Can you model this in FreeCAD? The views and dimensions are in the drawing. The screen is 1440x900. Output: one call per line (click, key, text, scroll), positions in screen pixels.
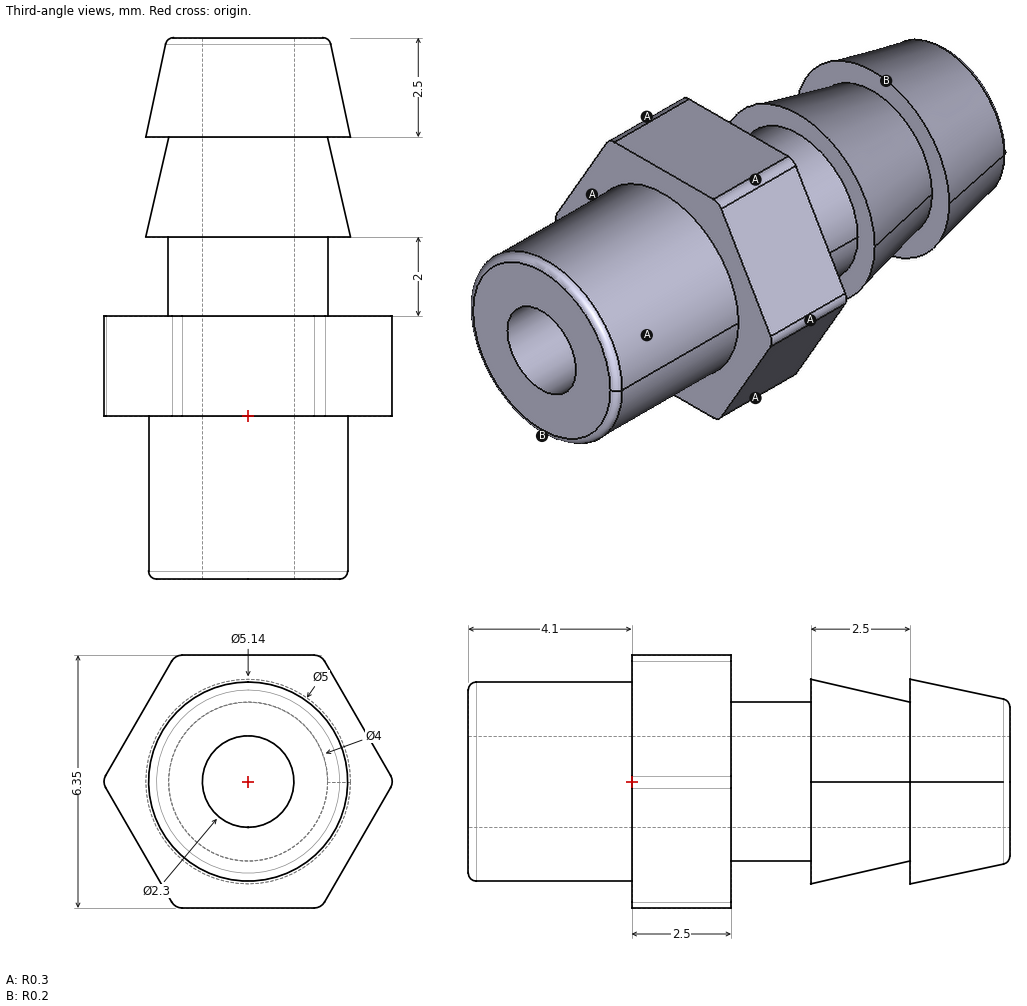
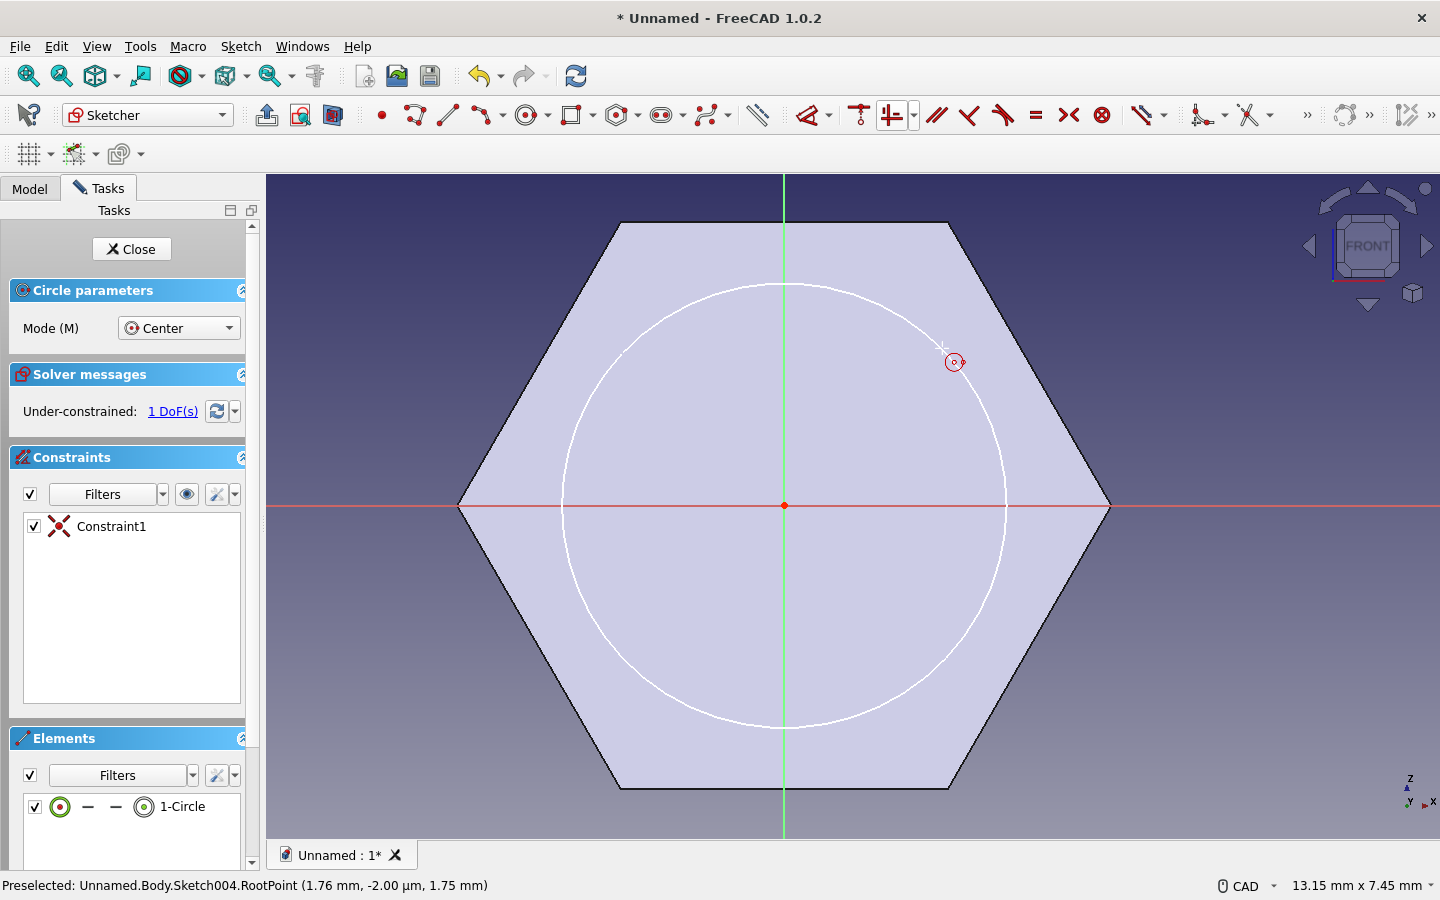
click(784, 506)
click(857, 433)
key(Escape)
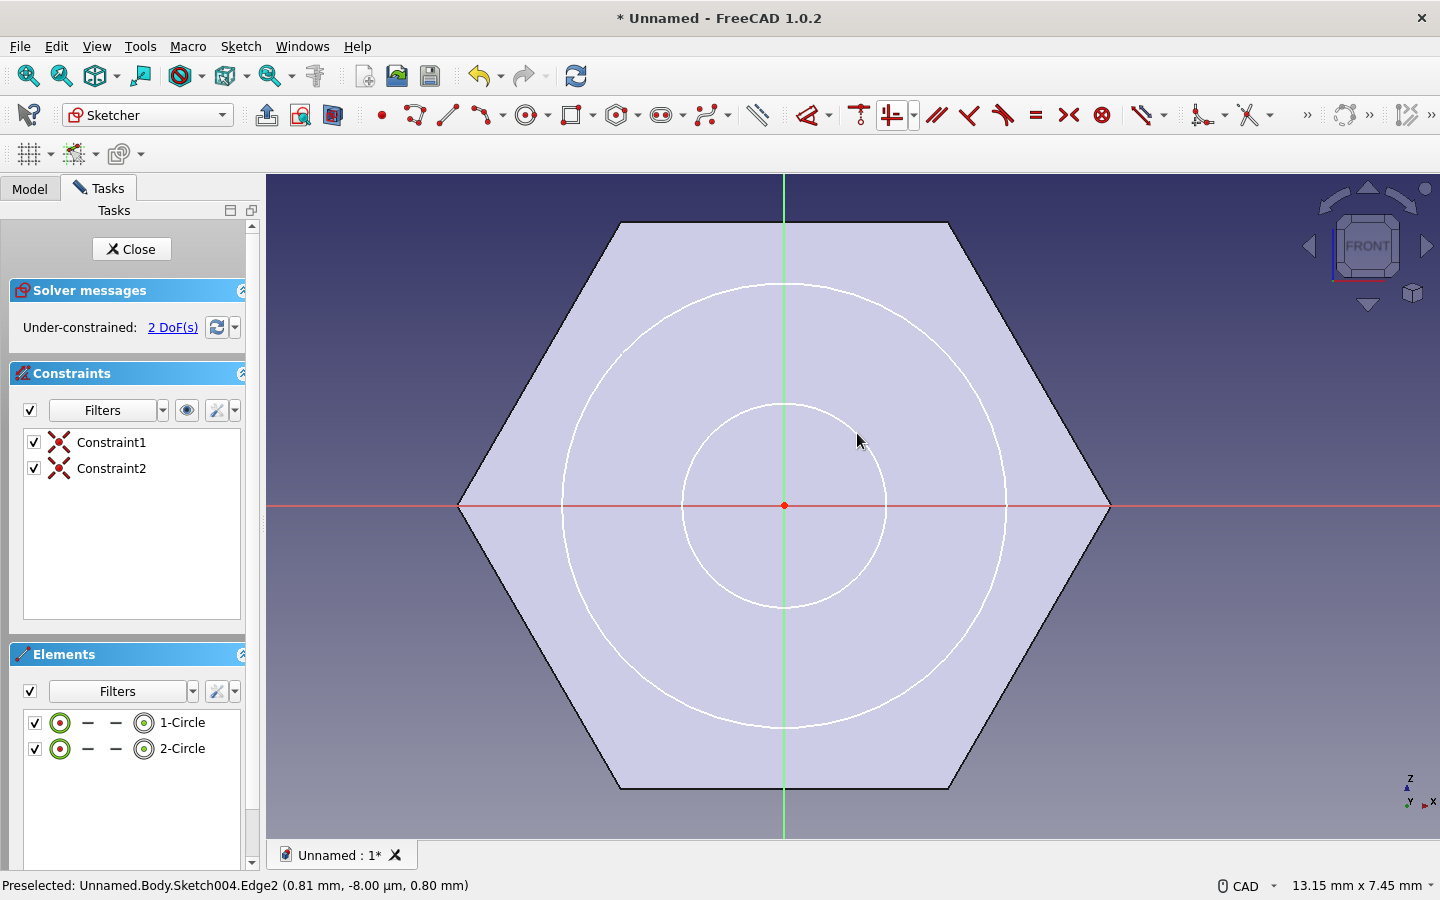
click(806, 116)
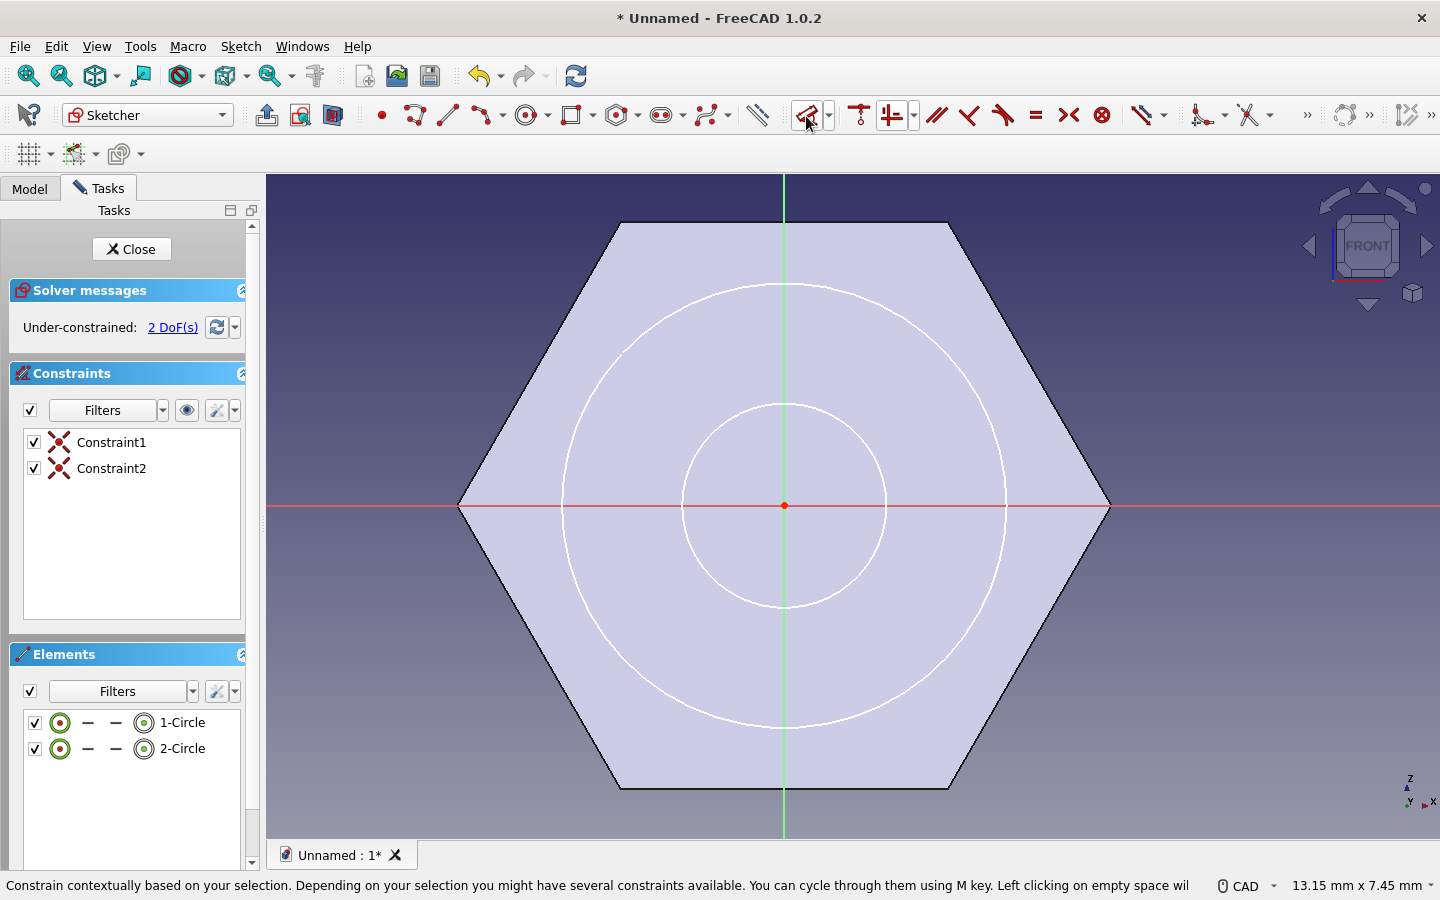
click(941, 348)
click(964, 325)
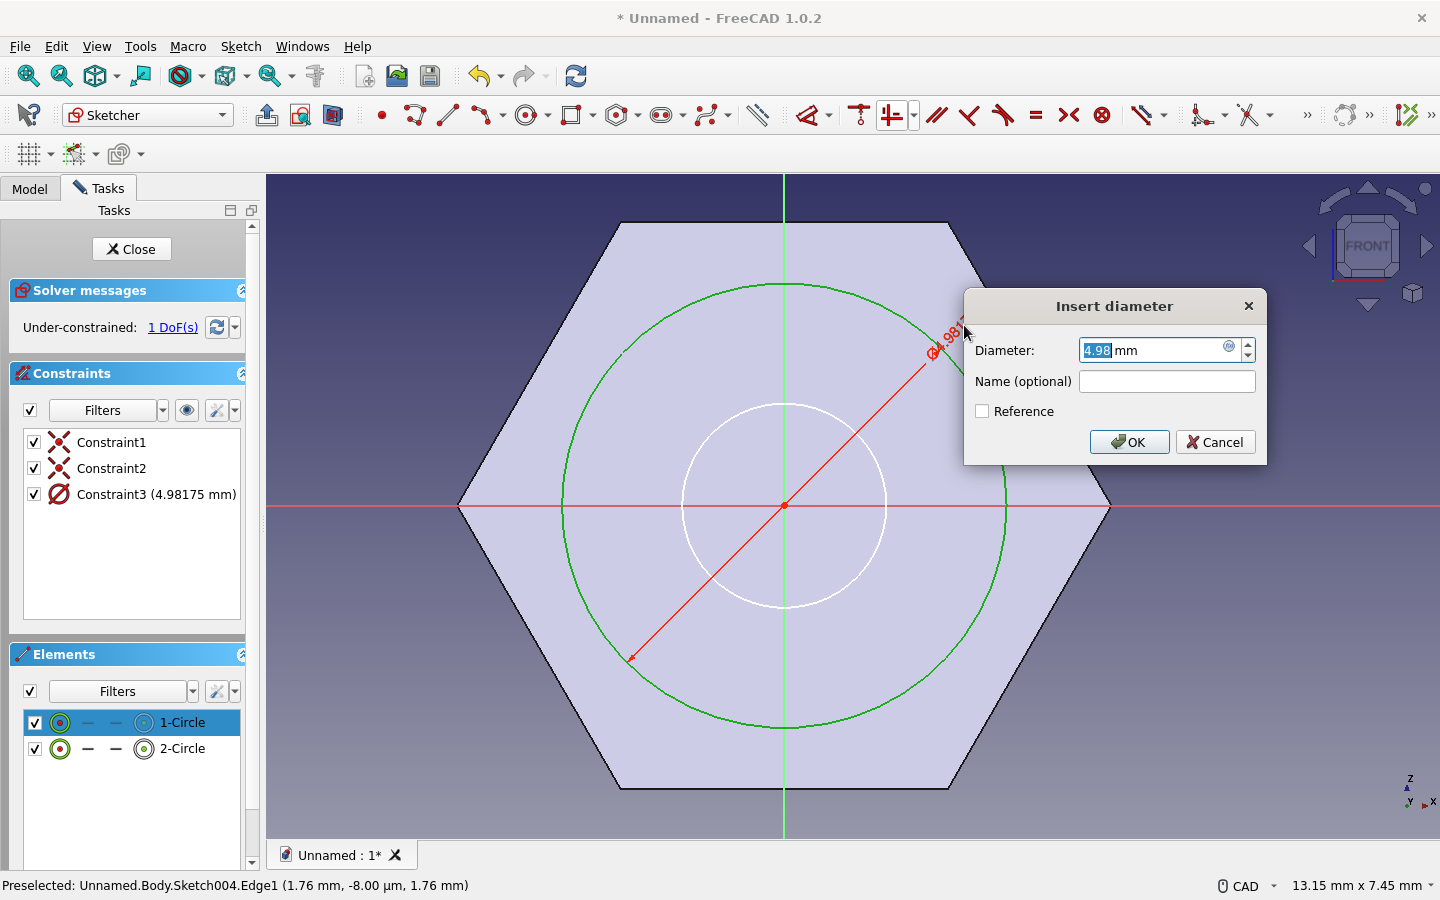
text(5)
key(Return)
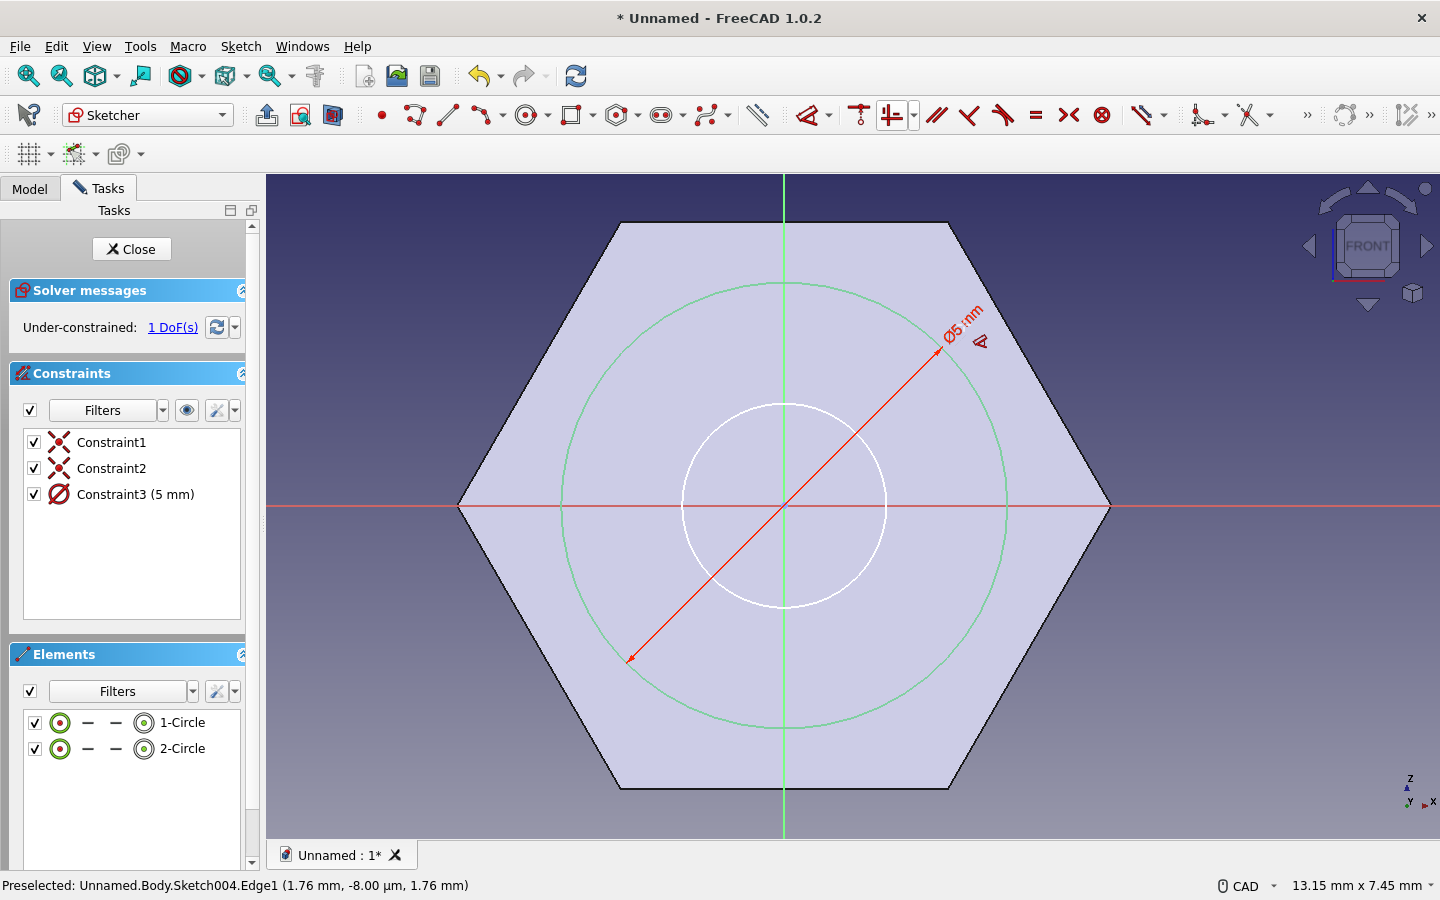
click(856, 433)
click(878, 410)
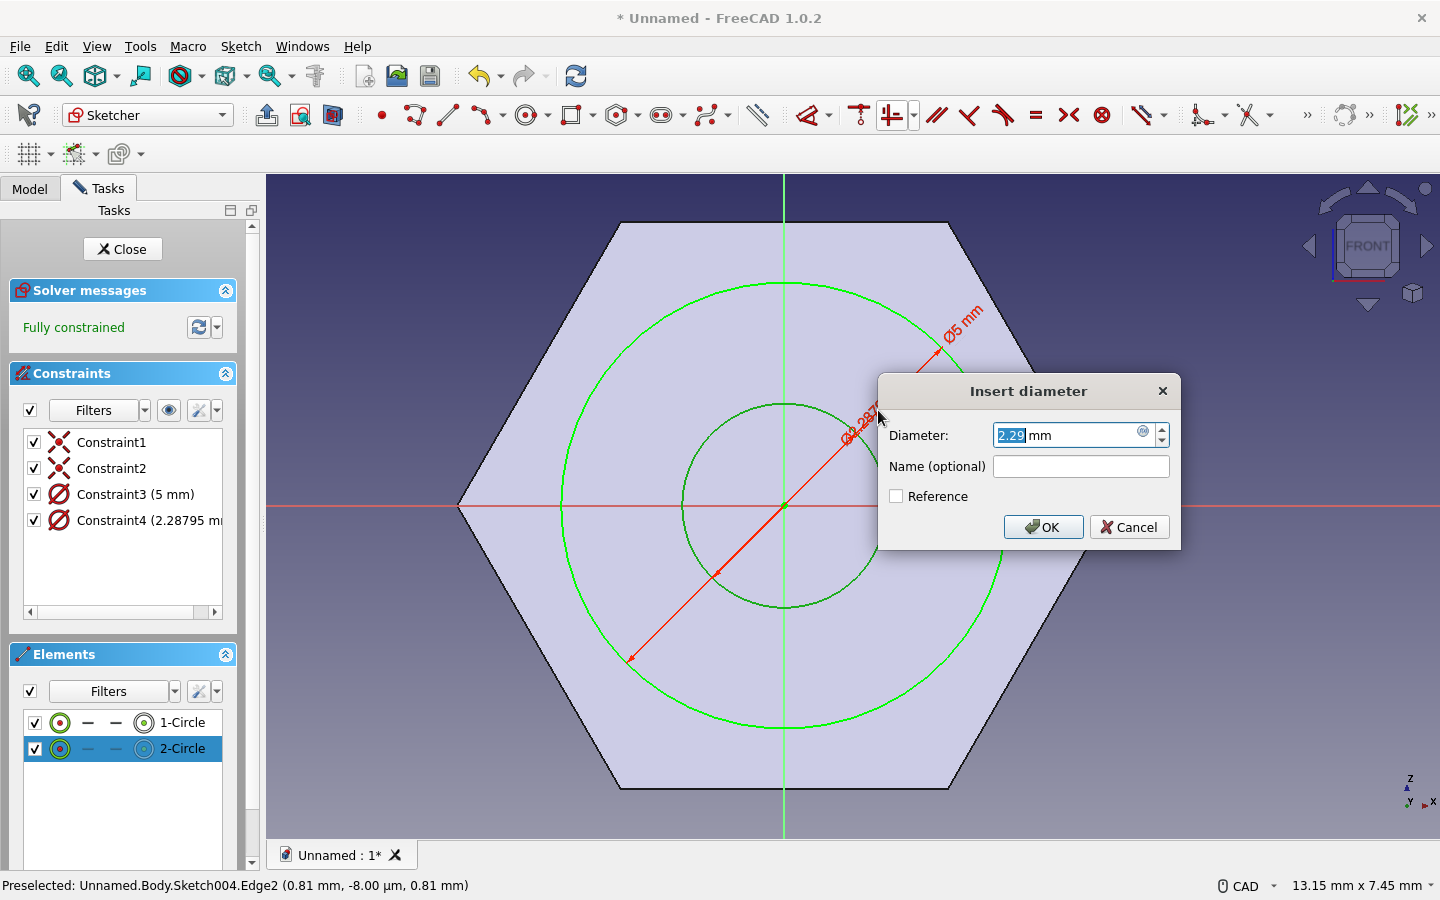
text(2.3)
key(Return)
key(Escape)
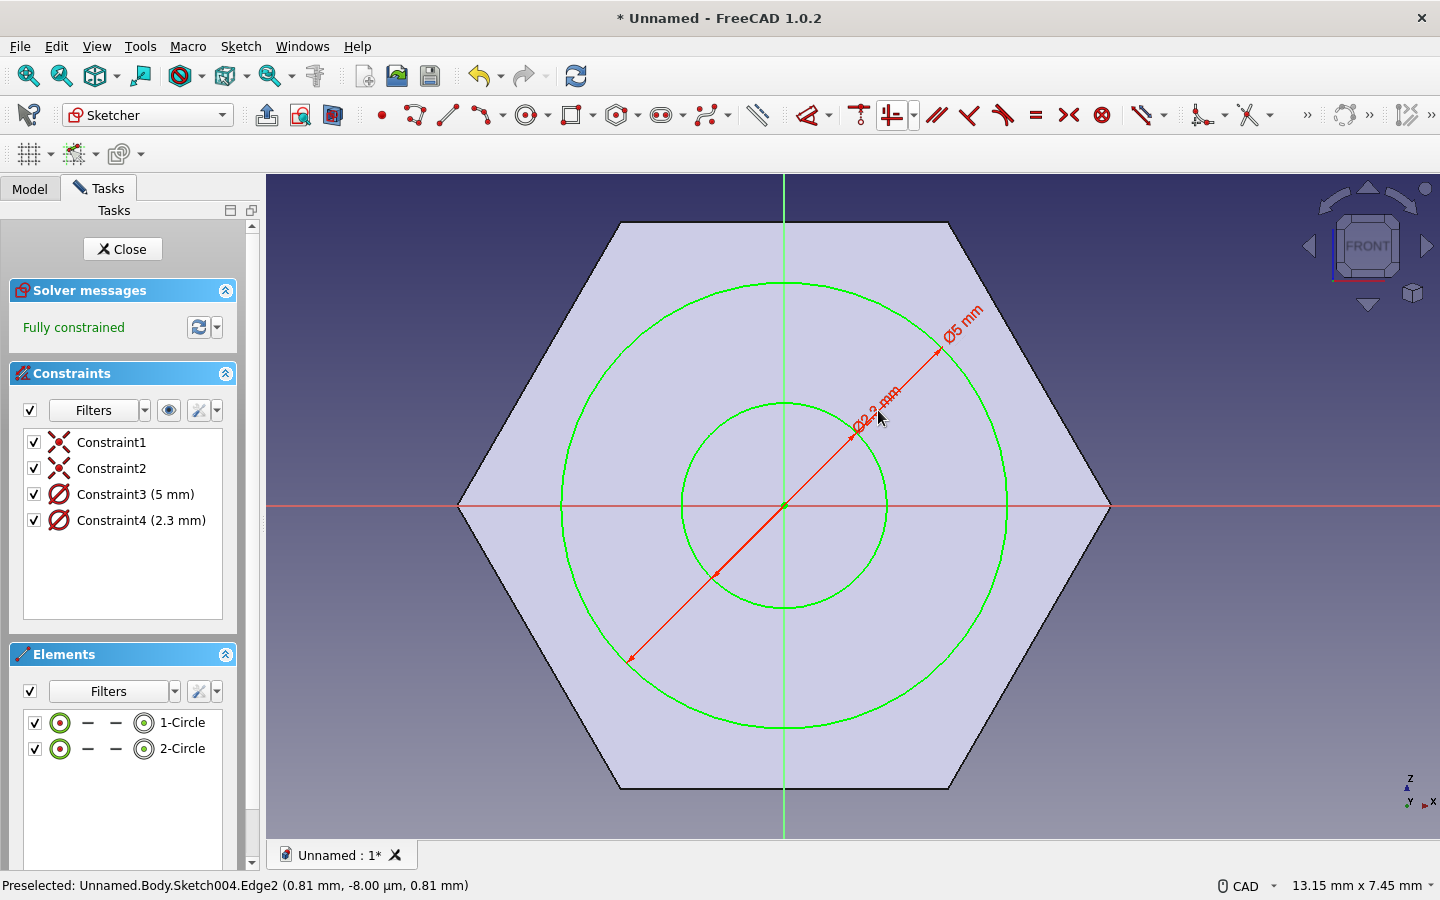
click(123, 249)